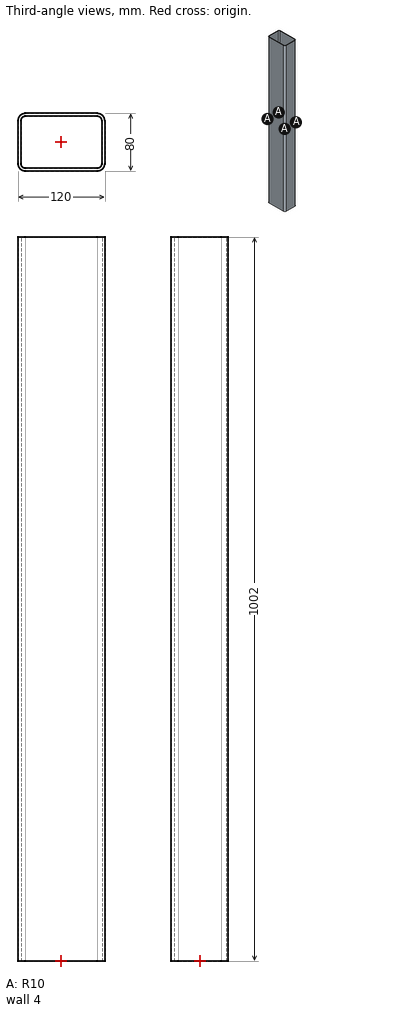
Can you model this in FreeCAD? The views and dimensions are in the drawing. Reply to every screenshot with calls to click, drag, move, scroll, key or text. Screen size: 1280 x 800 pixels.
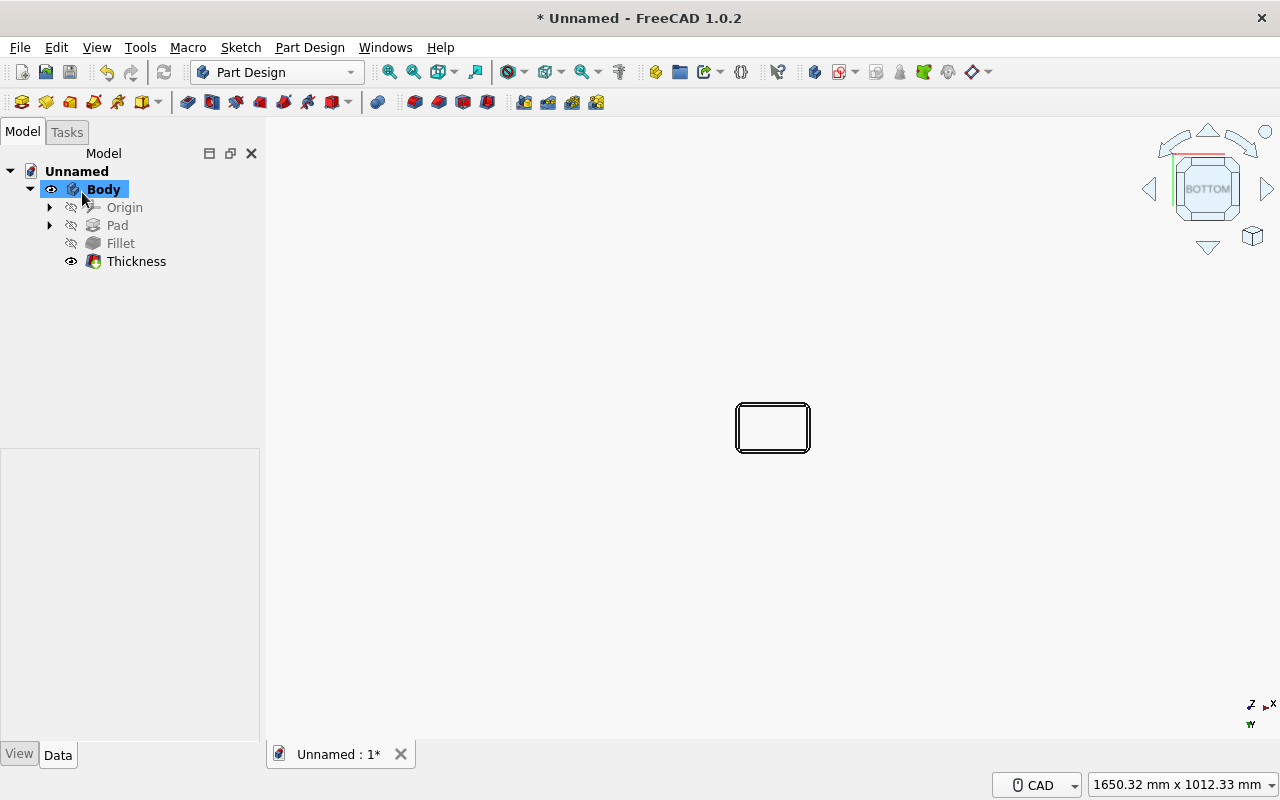
key(0)